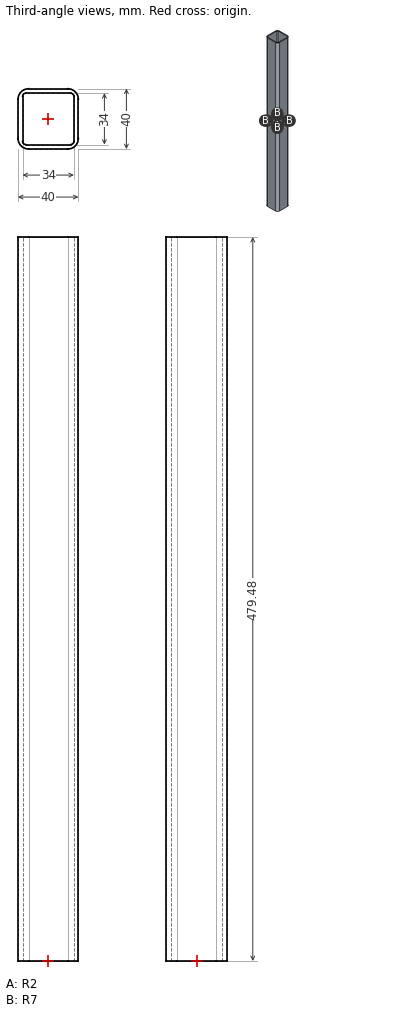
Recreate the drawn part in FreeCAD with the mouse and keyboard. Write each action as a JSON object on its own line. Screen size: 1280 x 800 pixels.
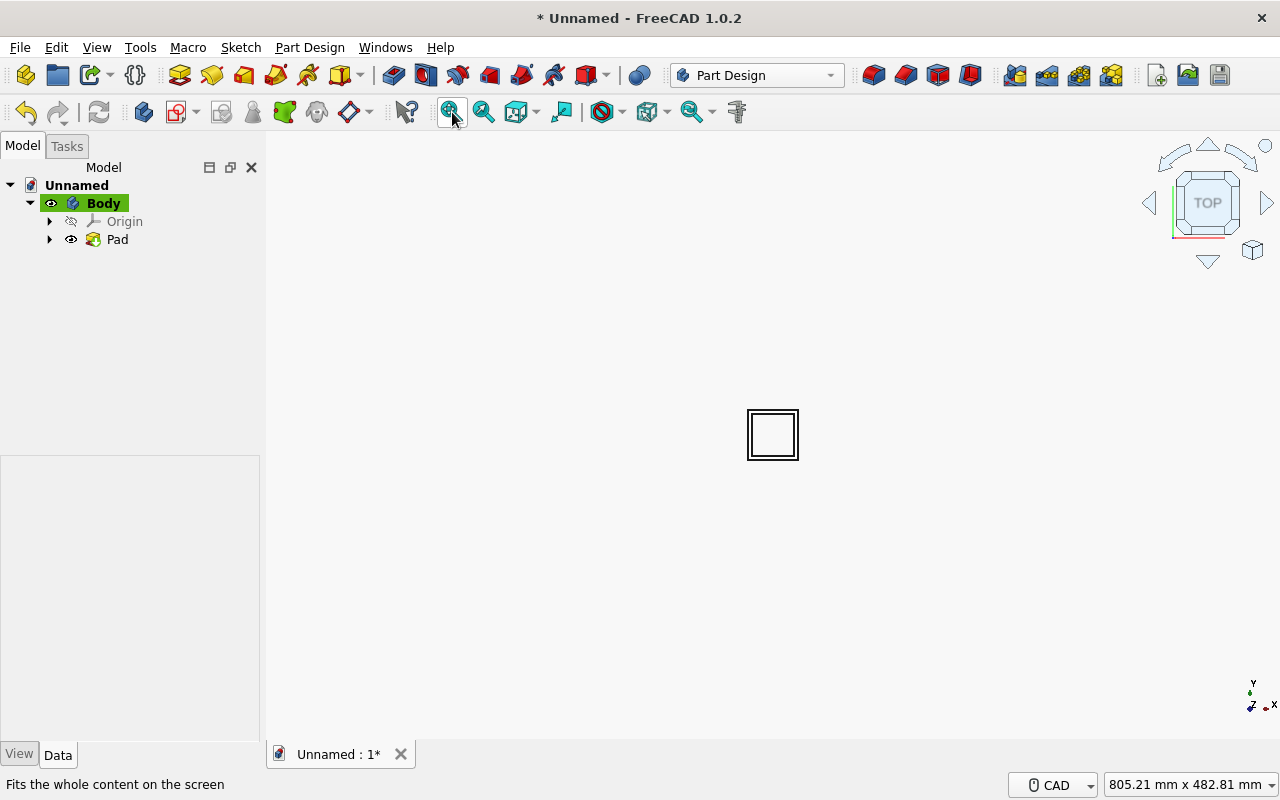
{"action": "key", "text": "1"}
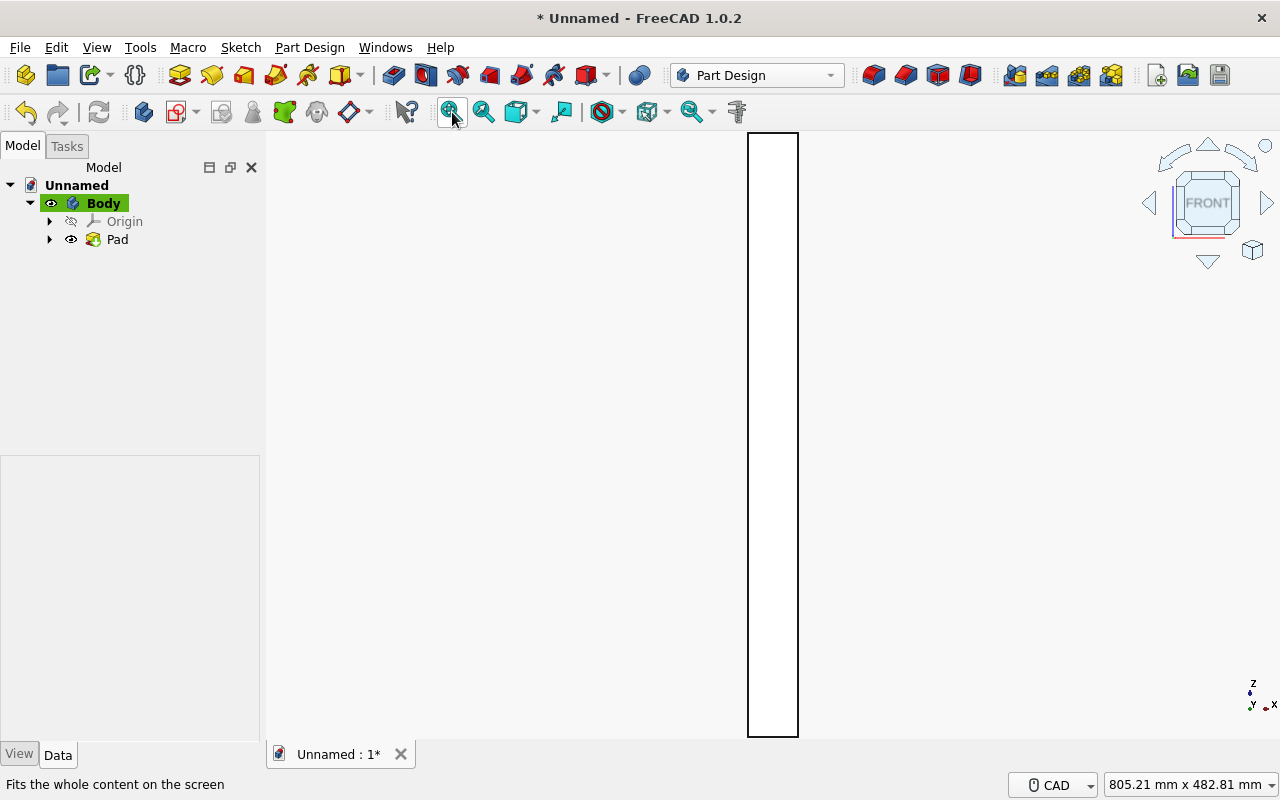
{"action": "key", "text": "3"}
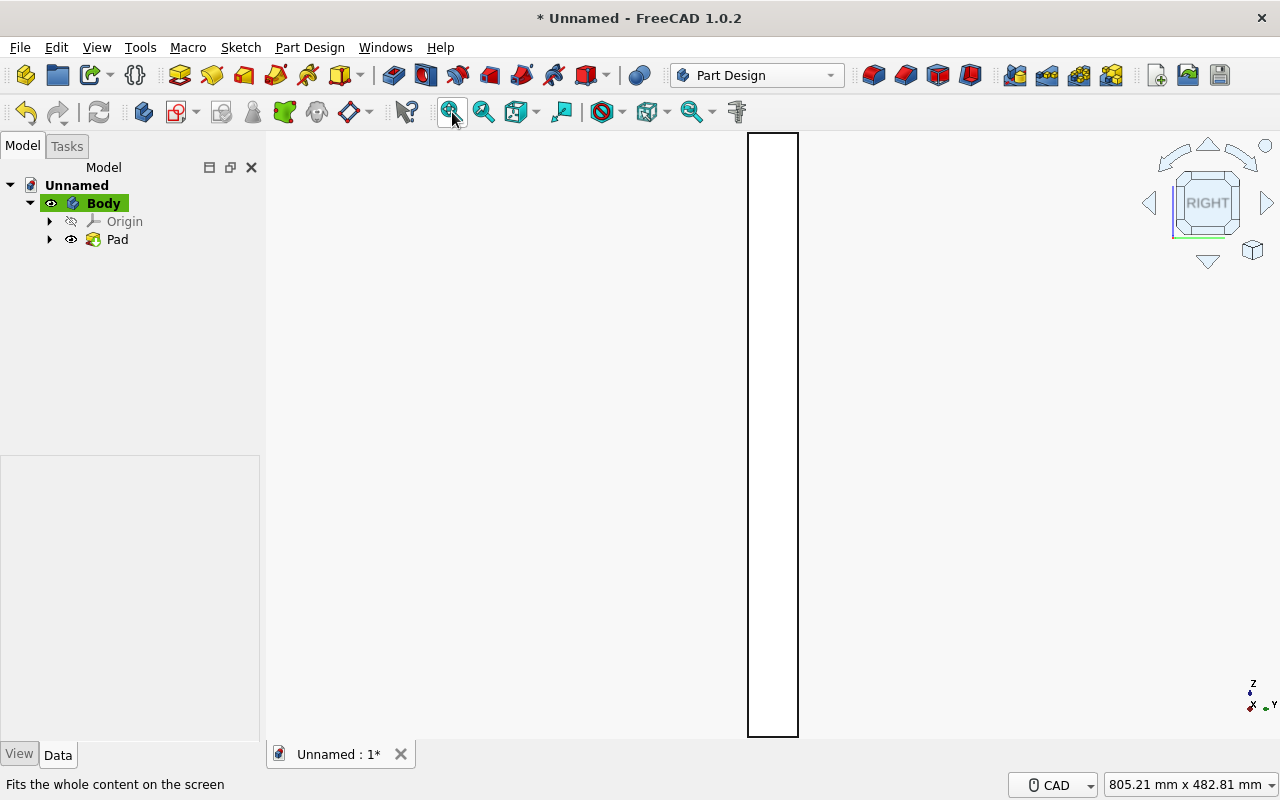
{"action": "key", "text": "5"}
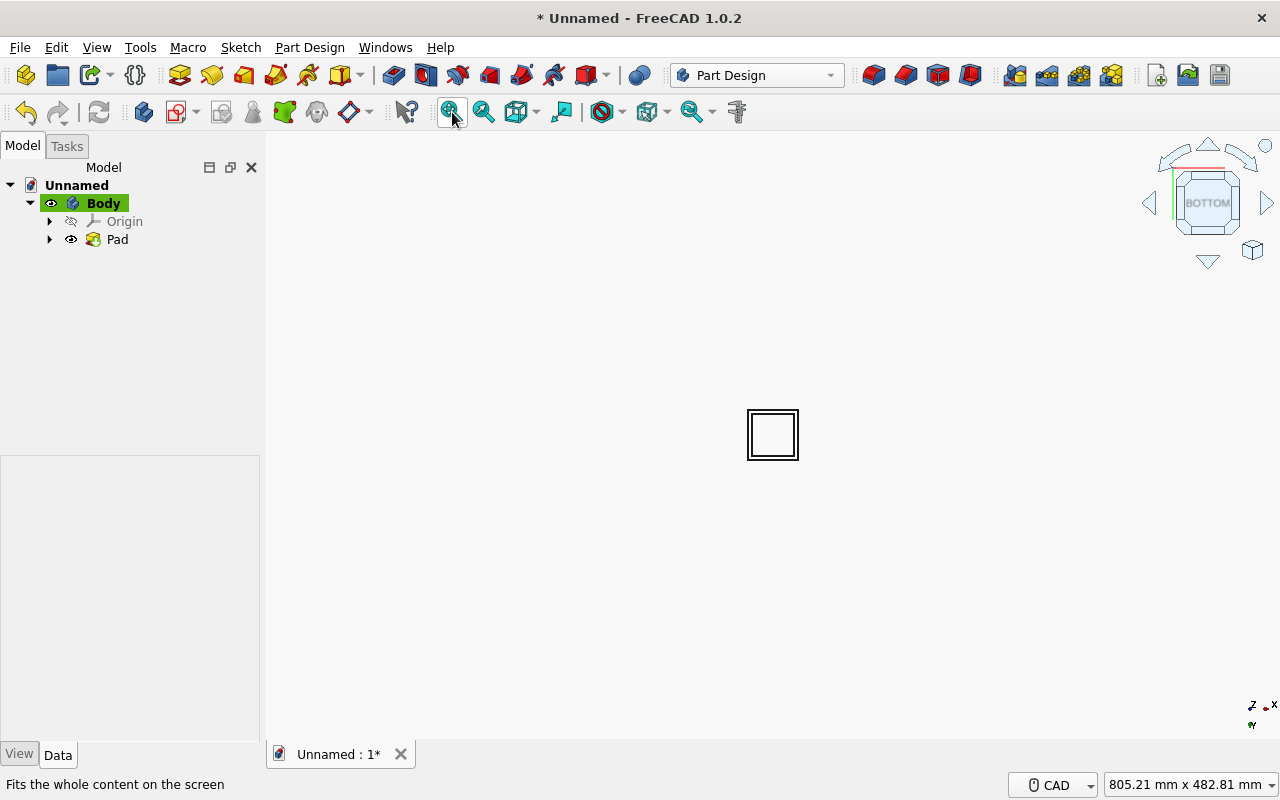
{"action": "key", "text": "v f"}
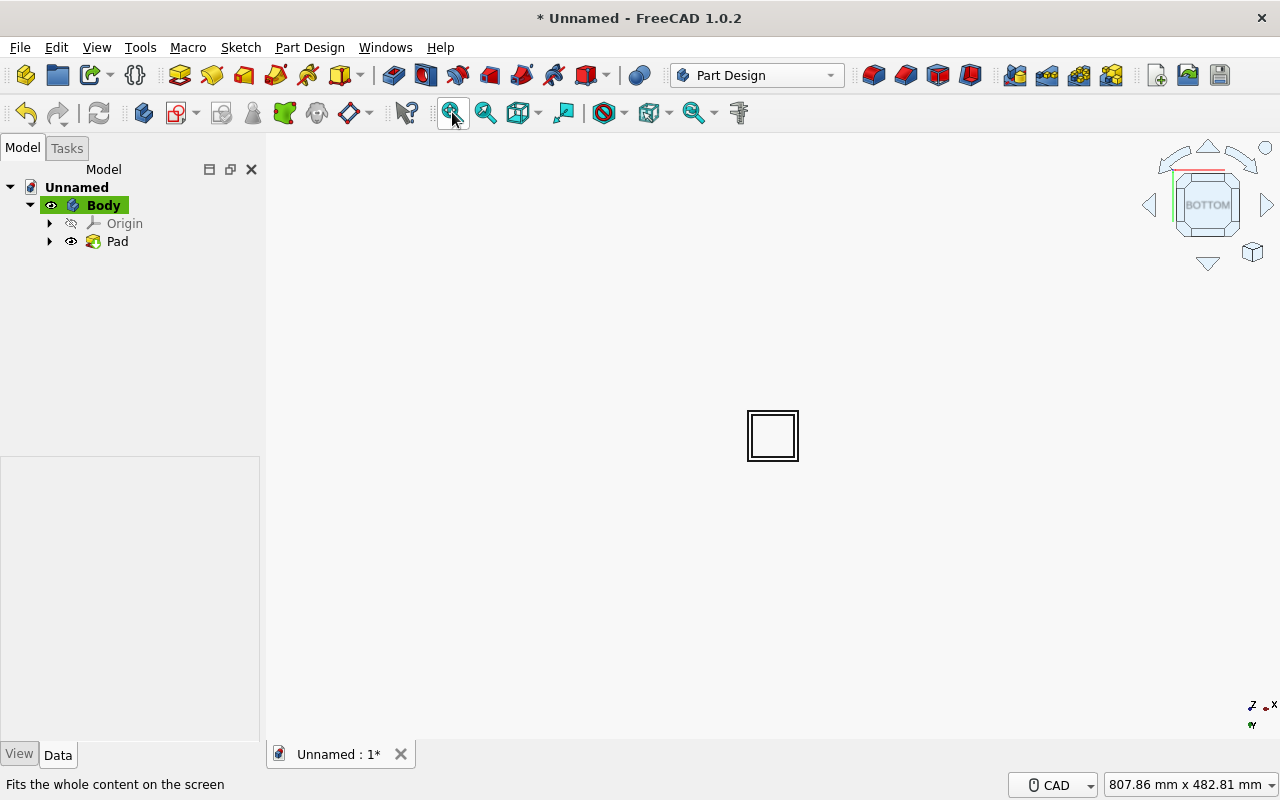
{"action": "key", "text": "4"}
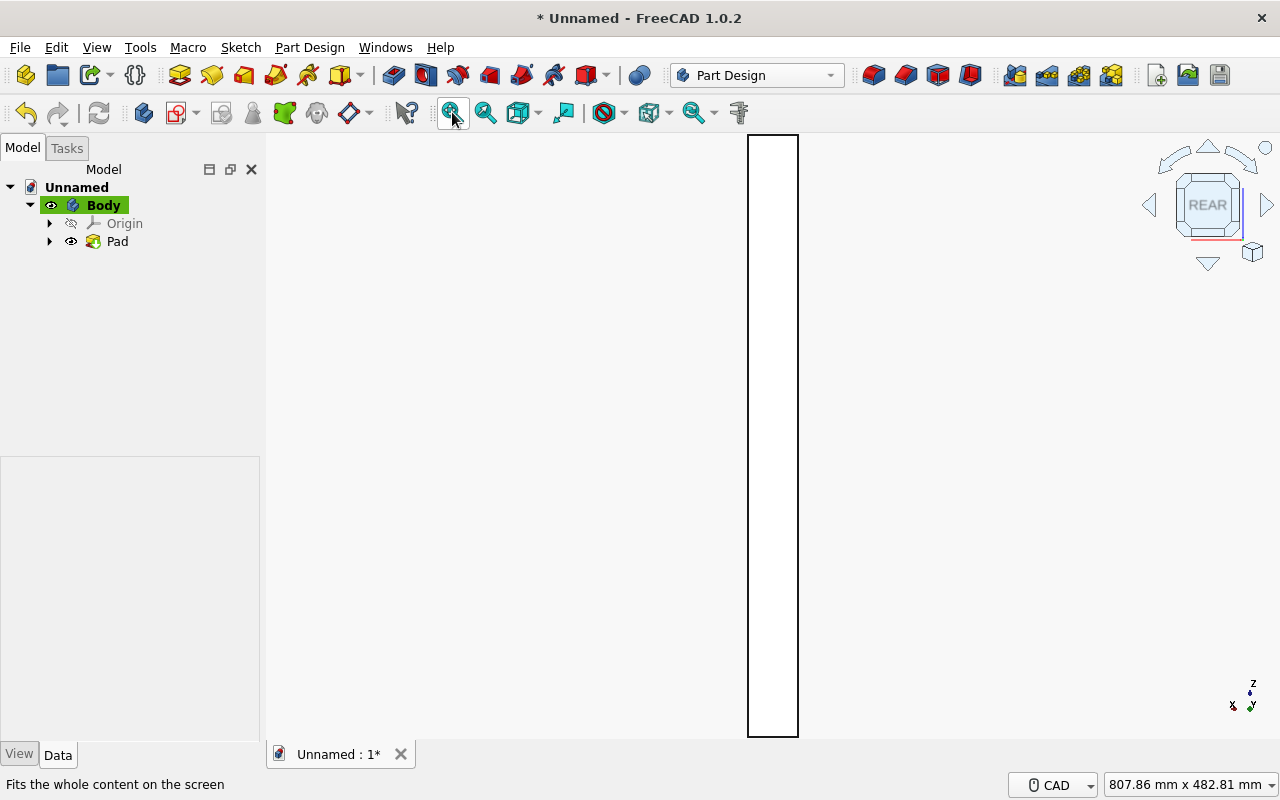
{"action": "key", "text": "6"}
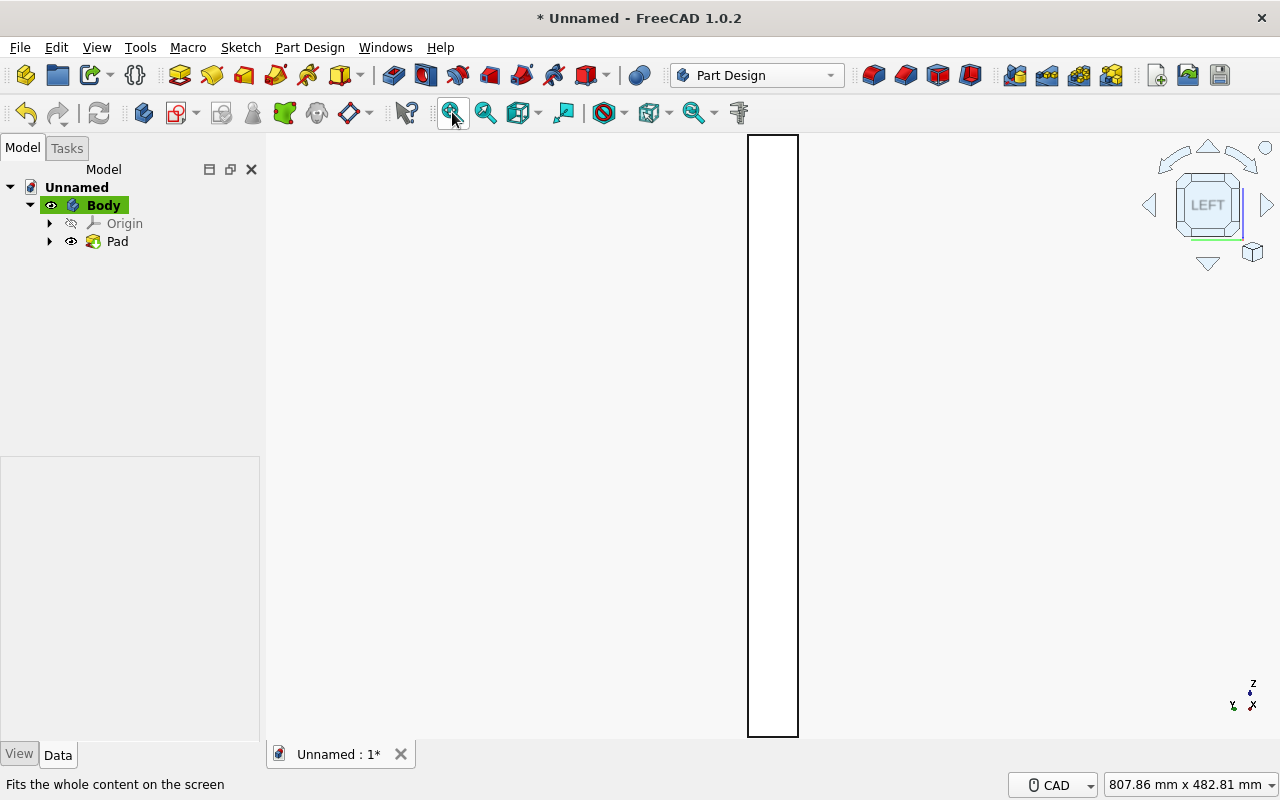
{"action": "key", "text": "v 3"}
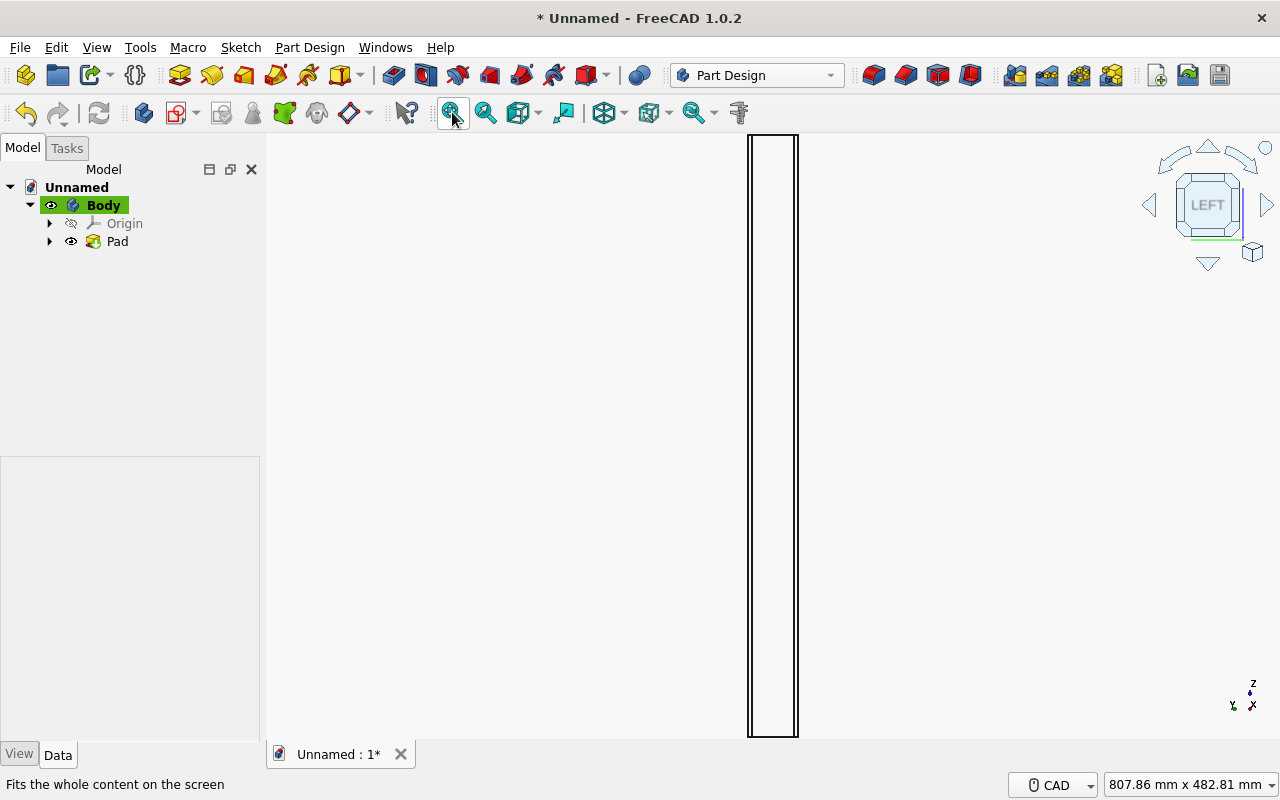
{"action": "key", "text": "0"}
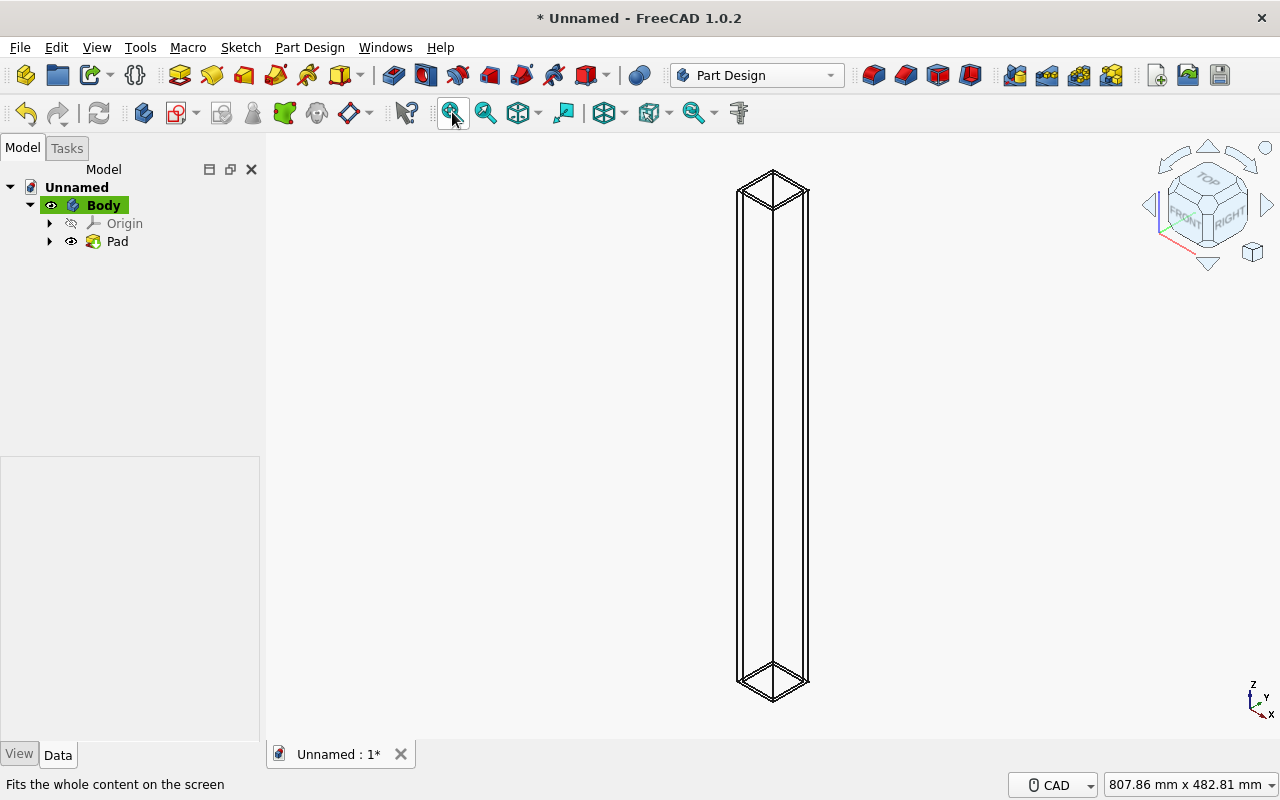
{"action": "left_click", "coordinate": [743, 435]}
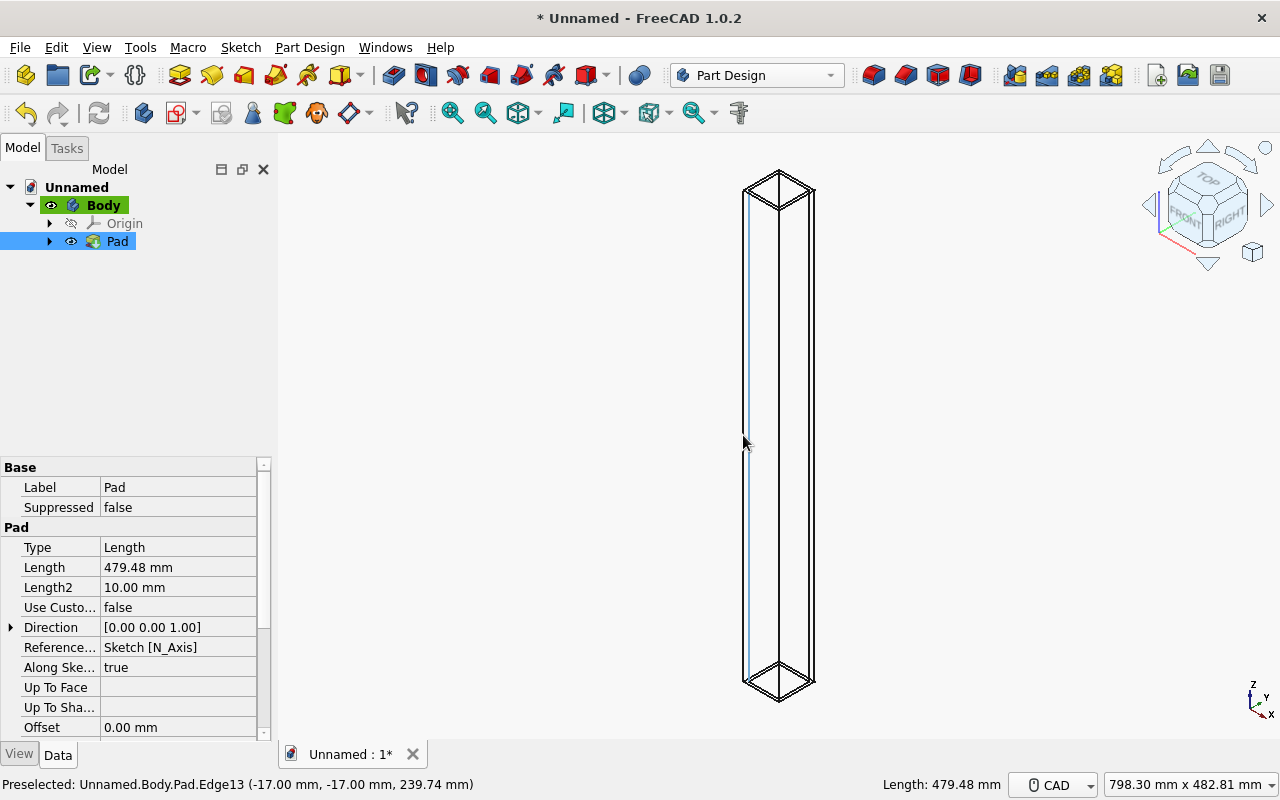
{"action": "scroll", "coordinate": [779, 452], "scroll_direction": "up", "scroll_amount": 6}